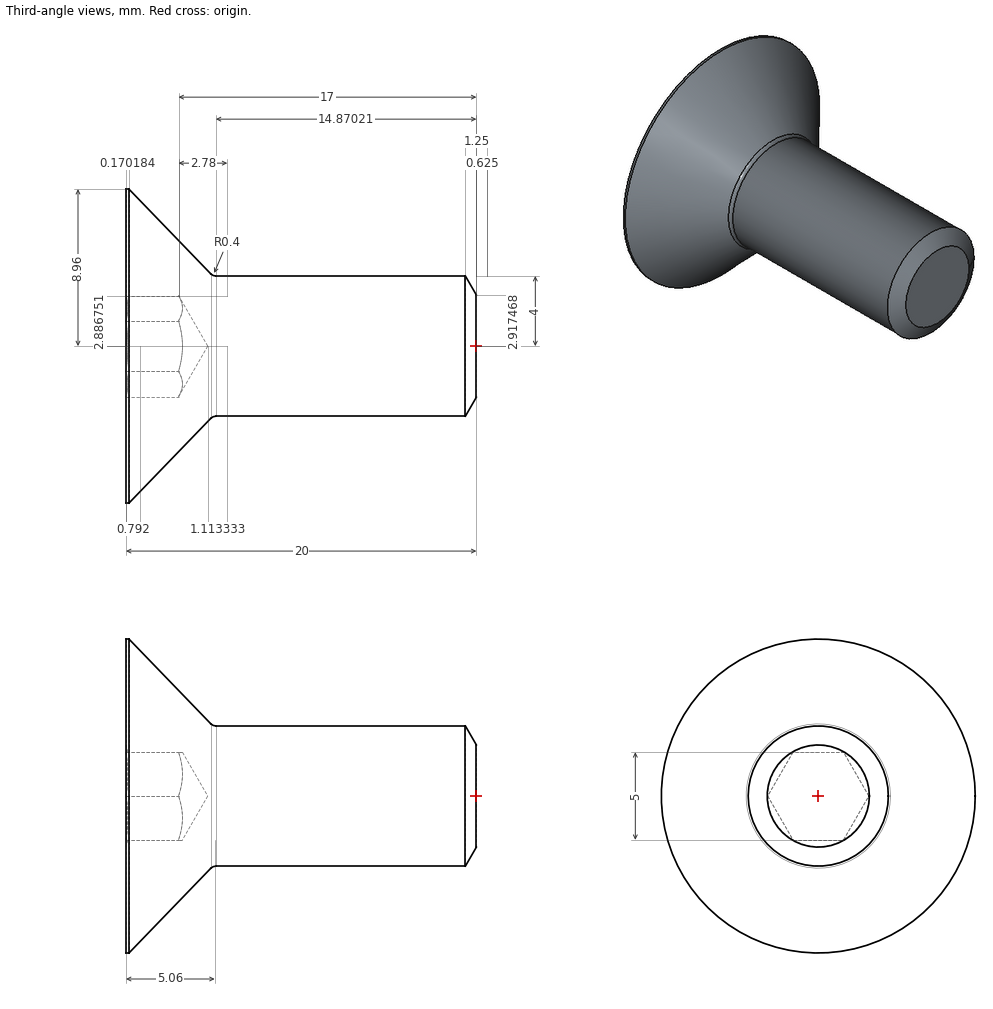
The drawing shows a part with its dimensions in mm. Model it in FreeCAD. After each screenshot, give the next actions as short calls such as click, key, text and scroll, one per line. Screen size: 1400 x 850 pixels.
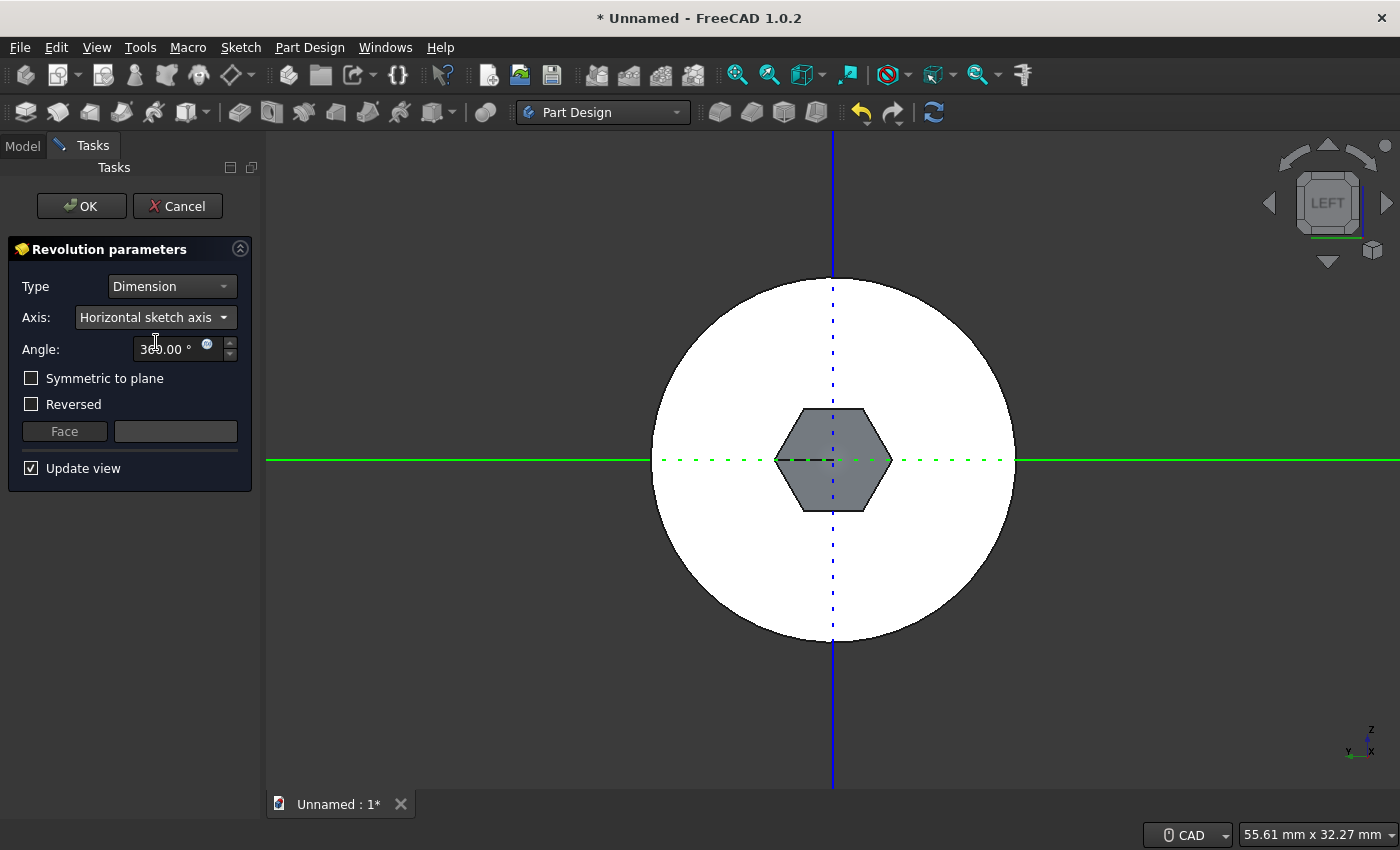
click(82, 206)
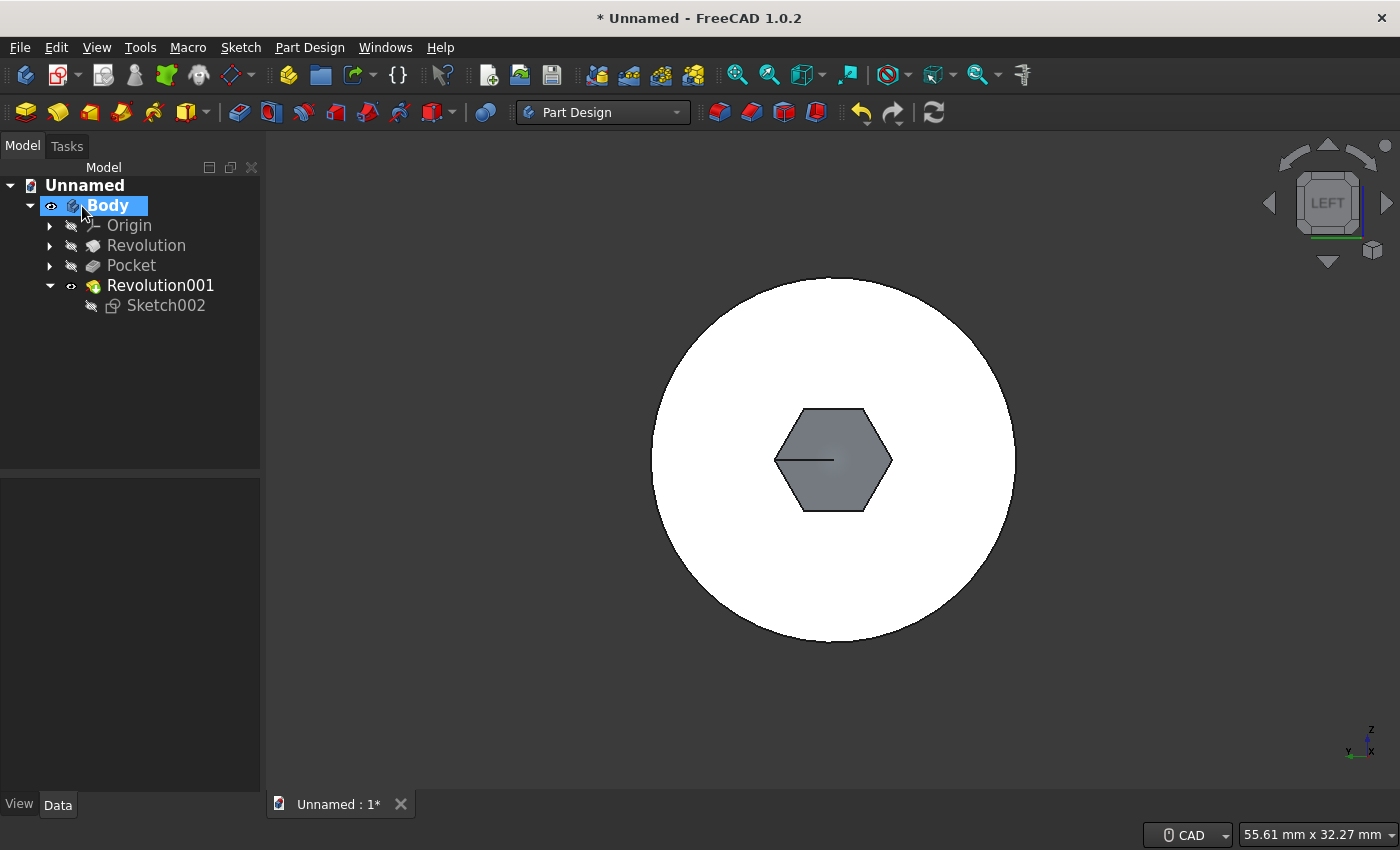
click(58, 76)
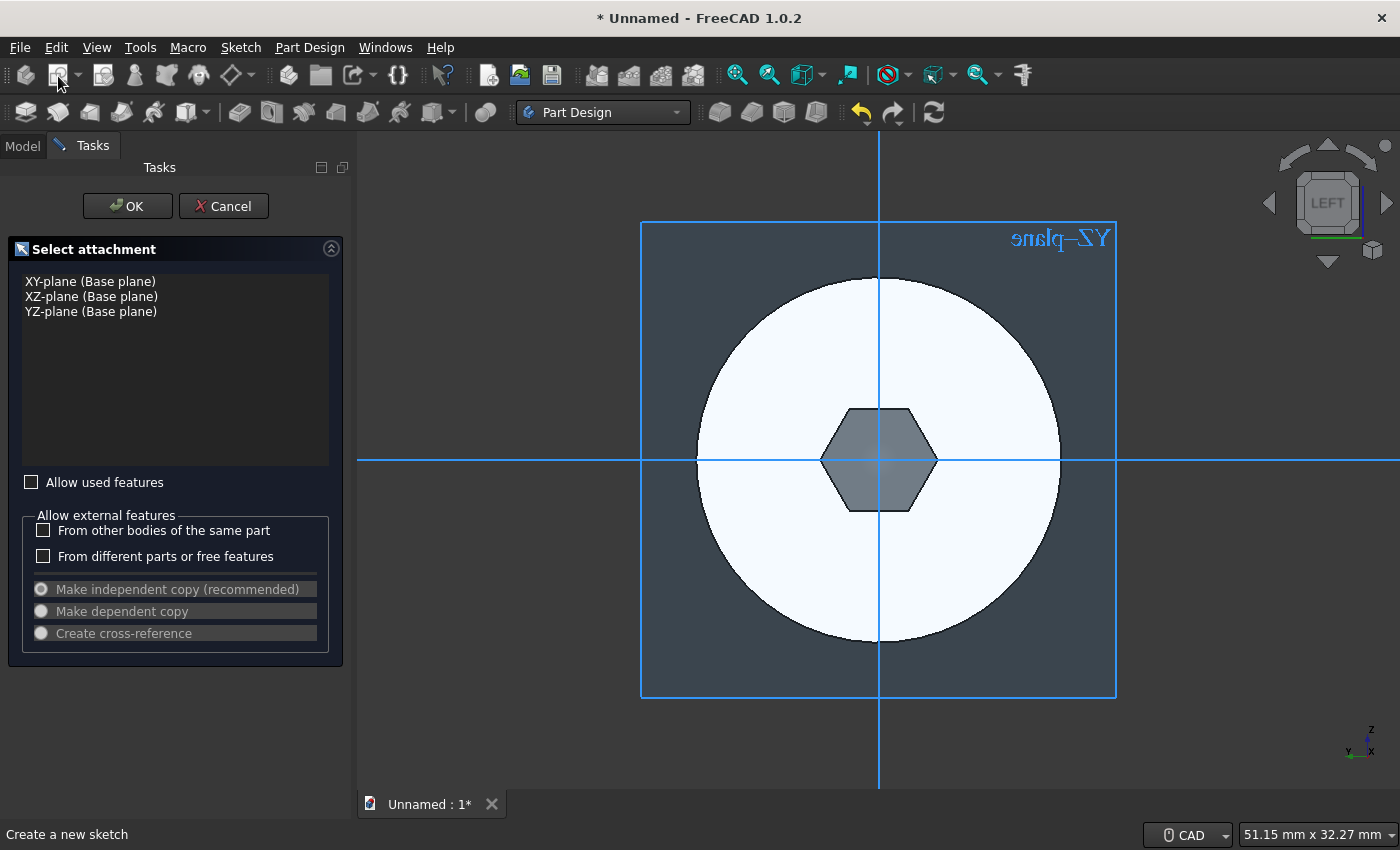
click(82, 282)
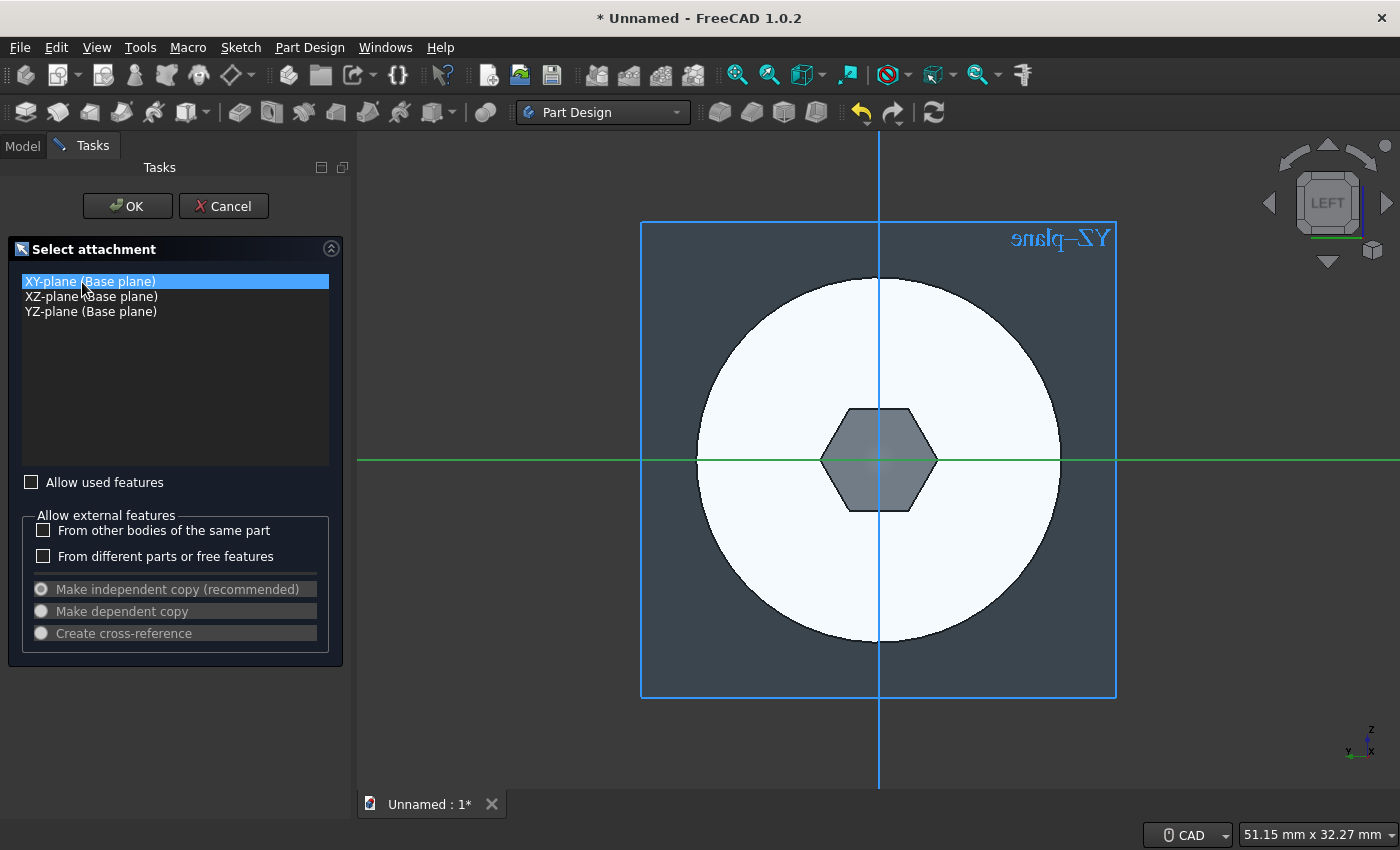
click(128, 206)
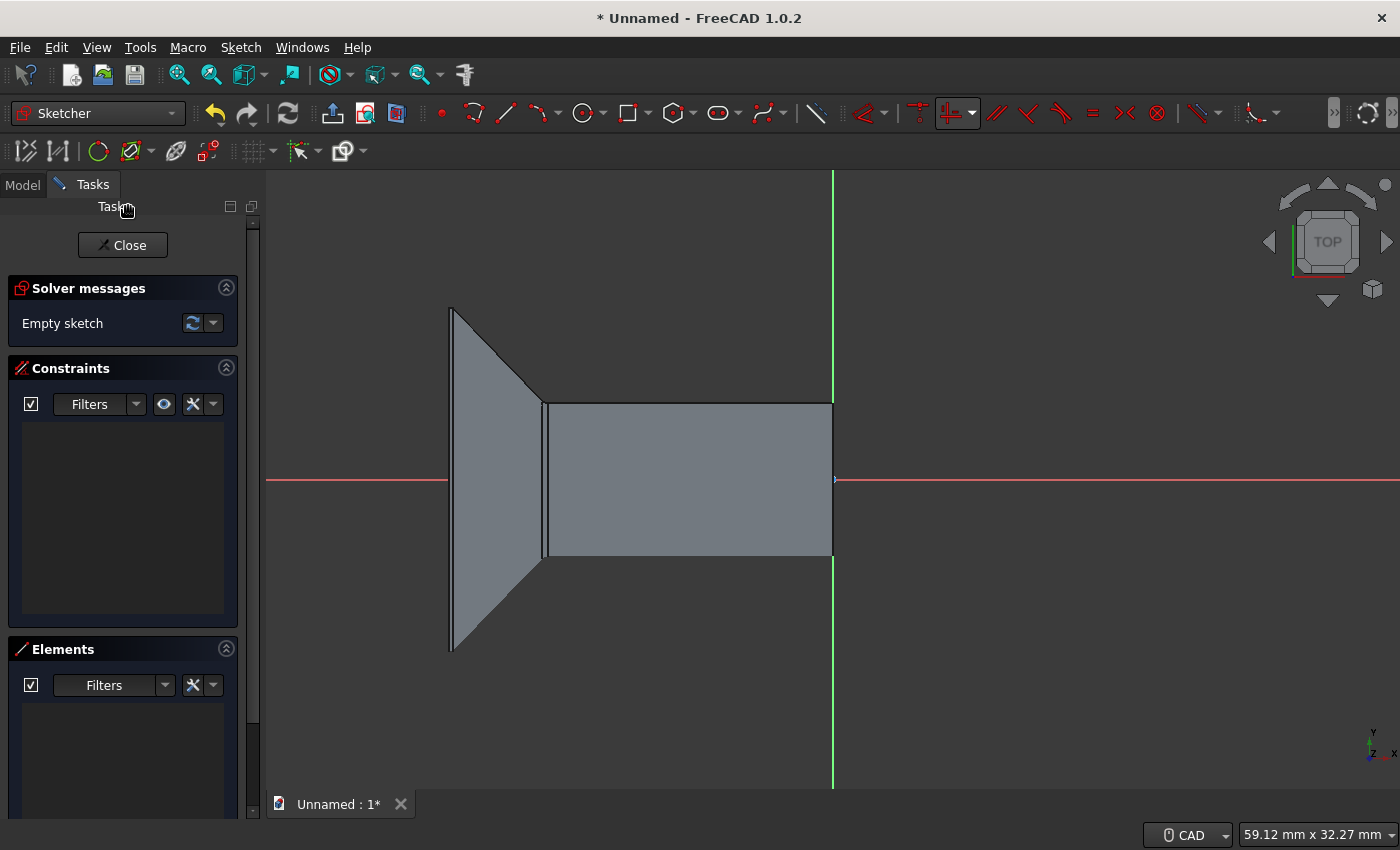
click(398, 114)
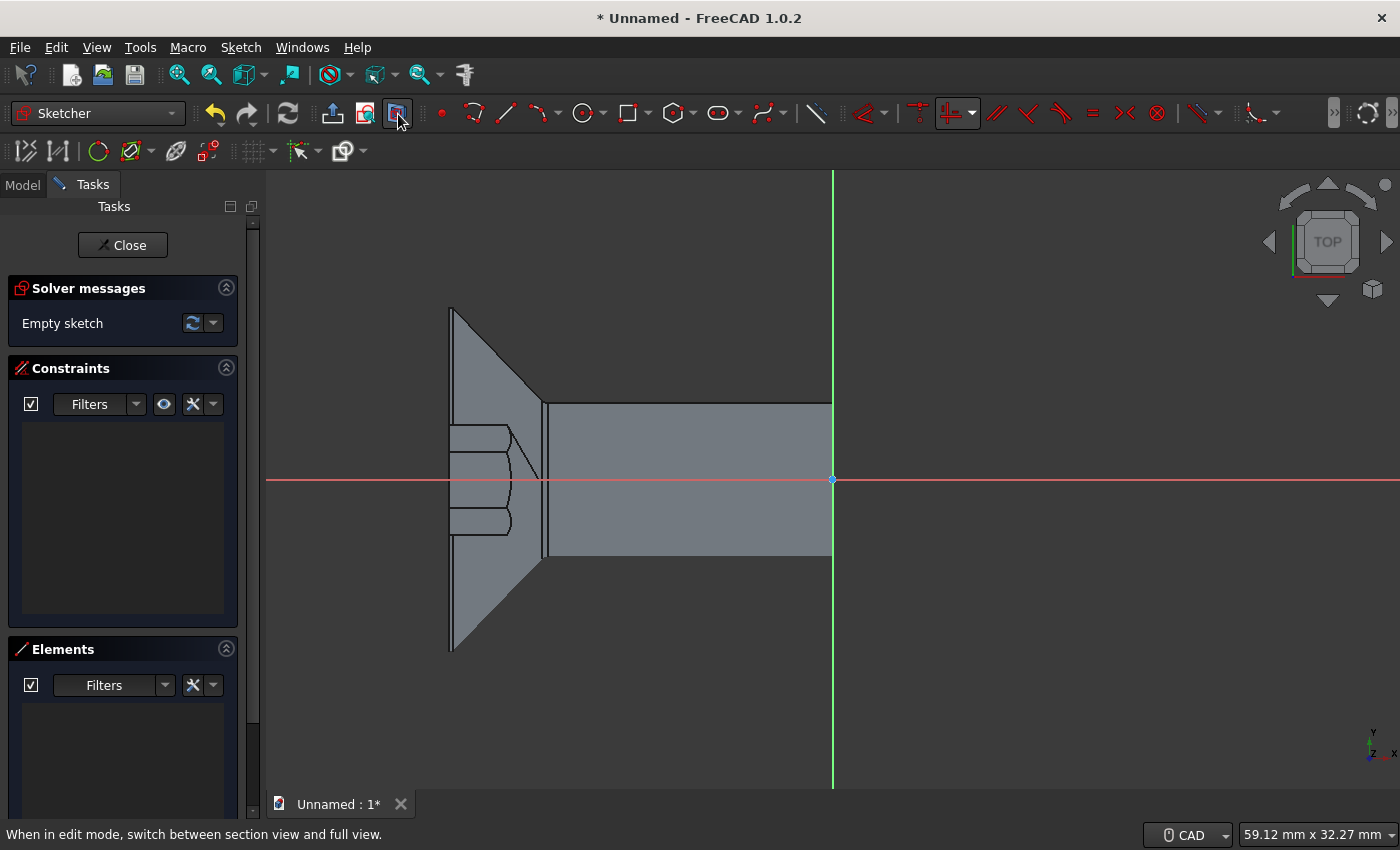
scroll(409, 448, up, 10)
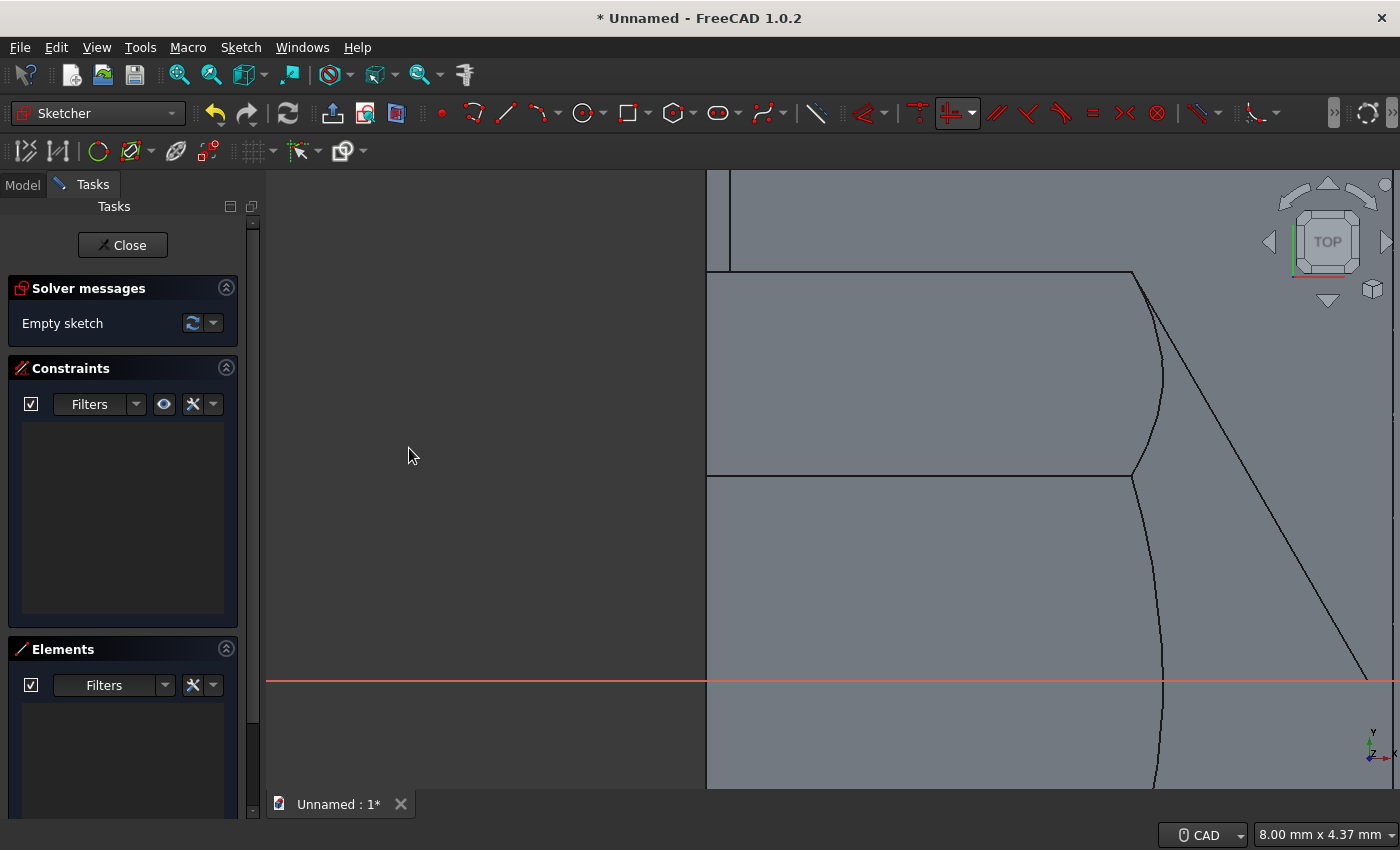
click(474, 114)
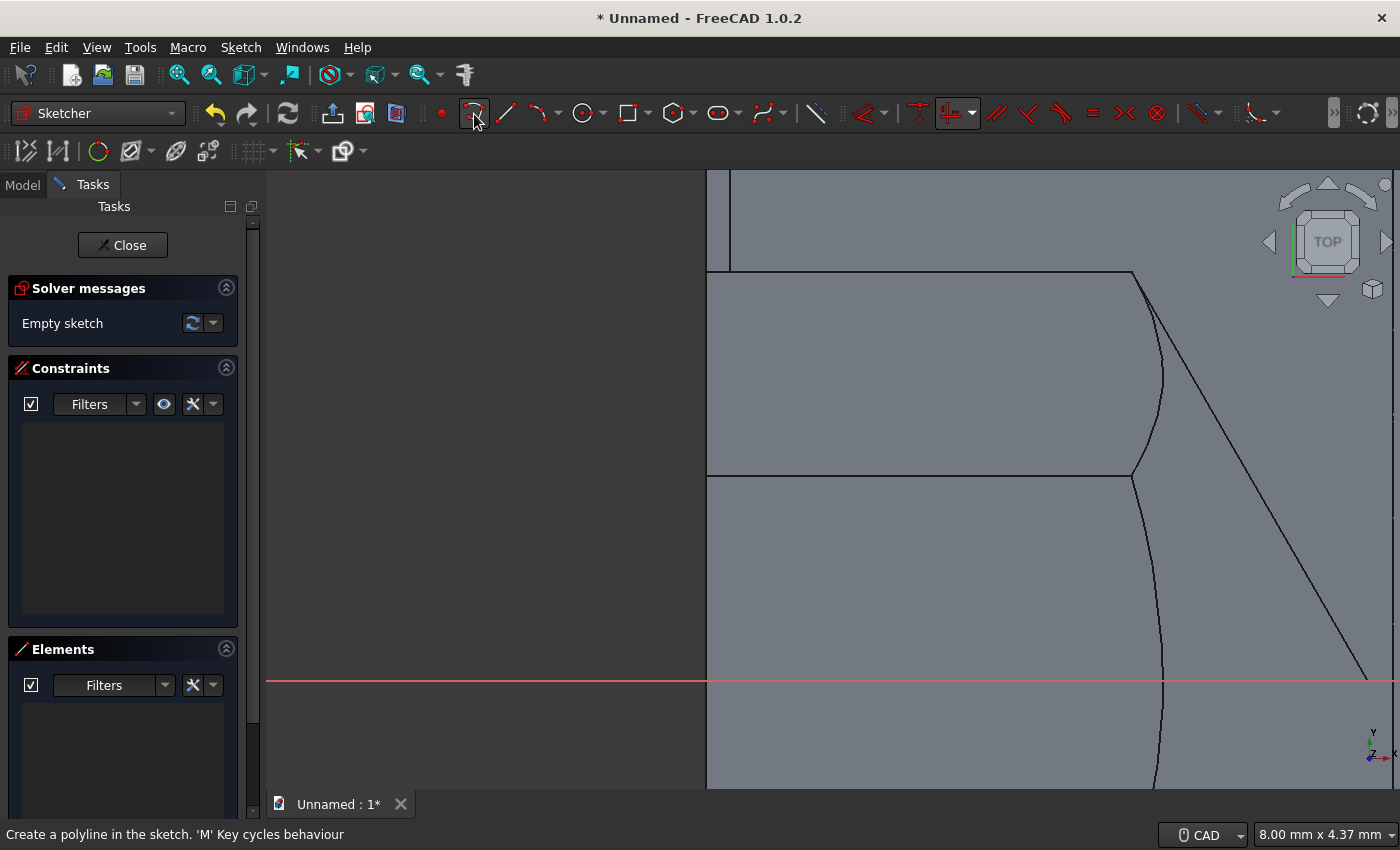
click(819, 681)
click(706, 272)
click(706, 672)
click(819, 681)
key(Escape)
key(Escape)